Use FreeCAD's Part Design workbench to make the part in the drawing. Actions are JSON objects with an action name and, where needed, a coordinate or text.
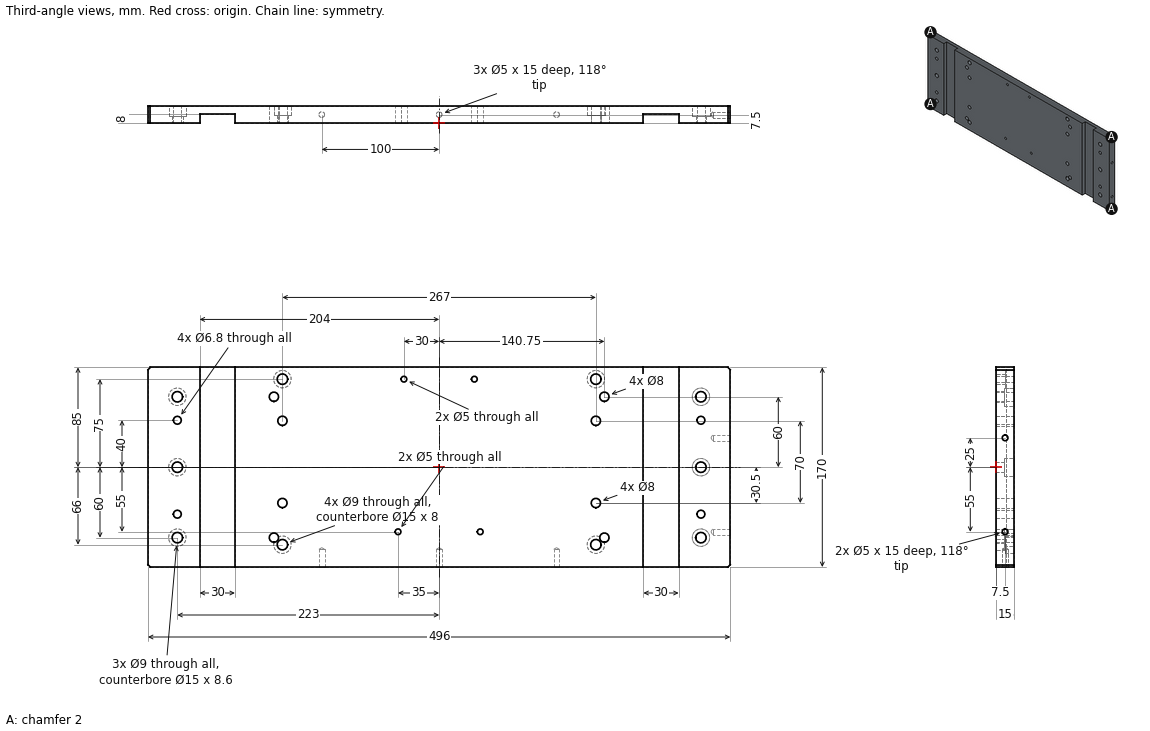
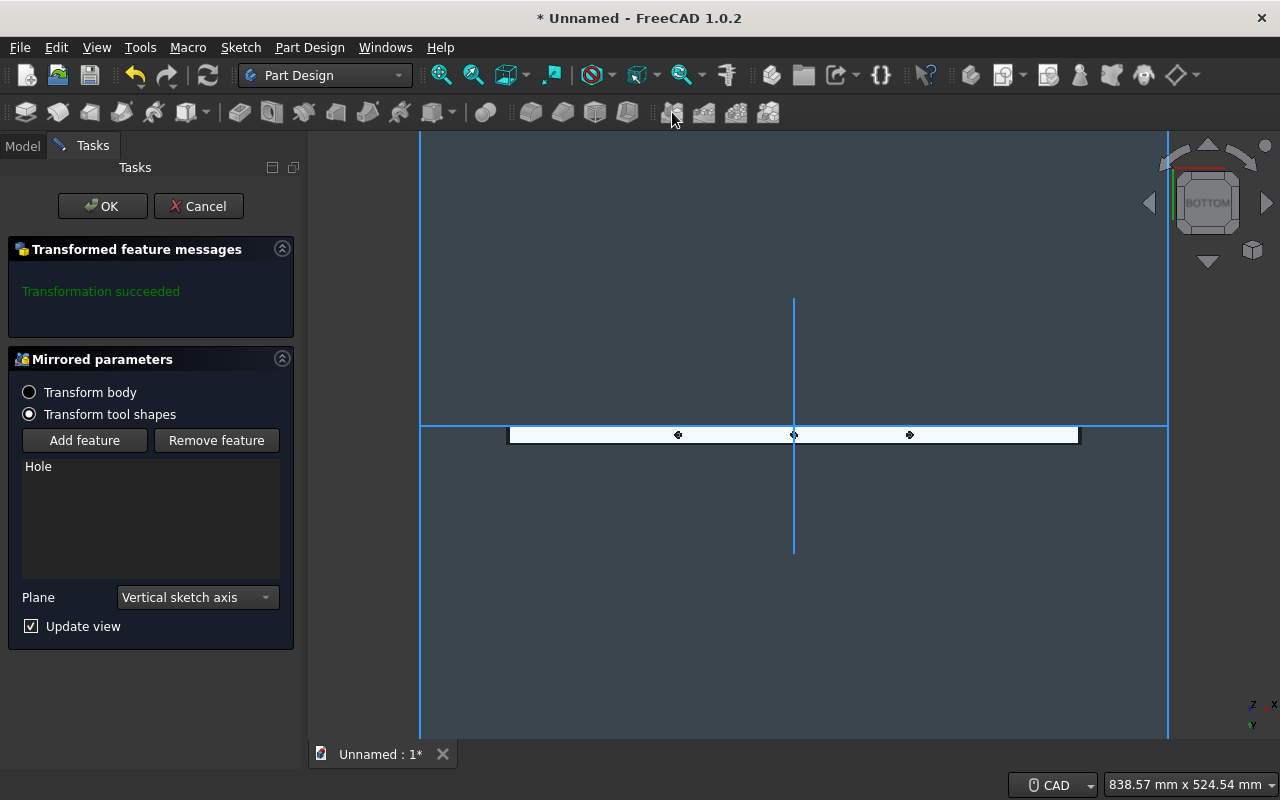
{"action": "left_click", "coordinate": [198, 598]}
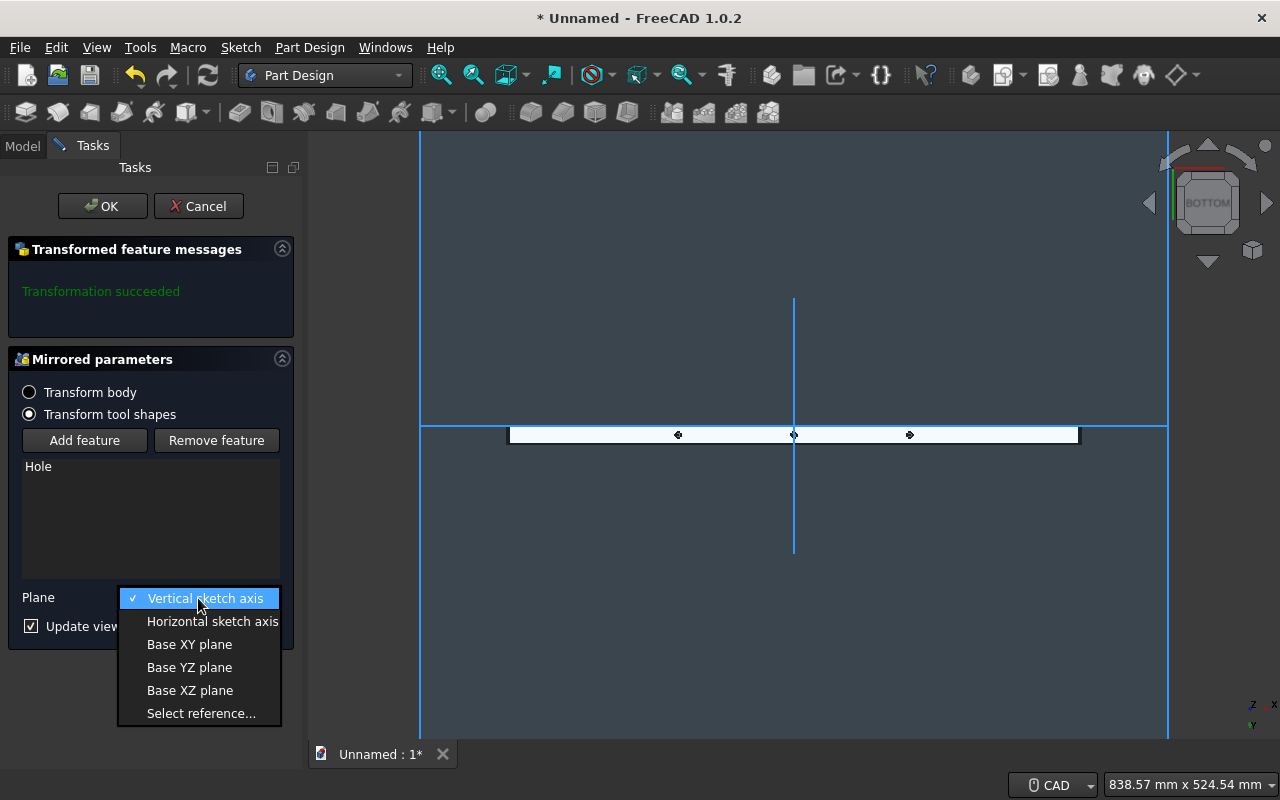
{"action": "left_click", "coordinate": [198, 668]}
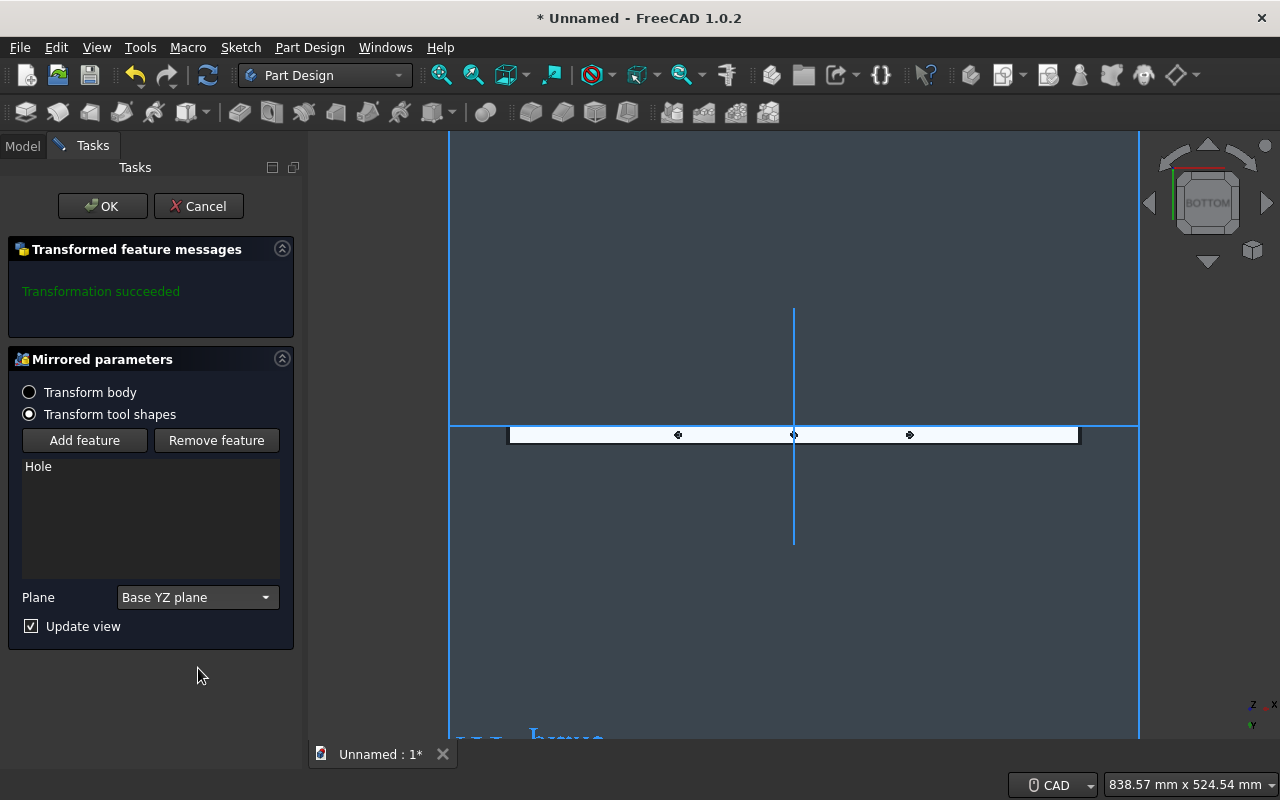
{"action": "left_click", "coordinate": [103, 206]}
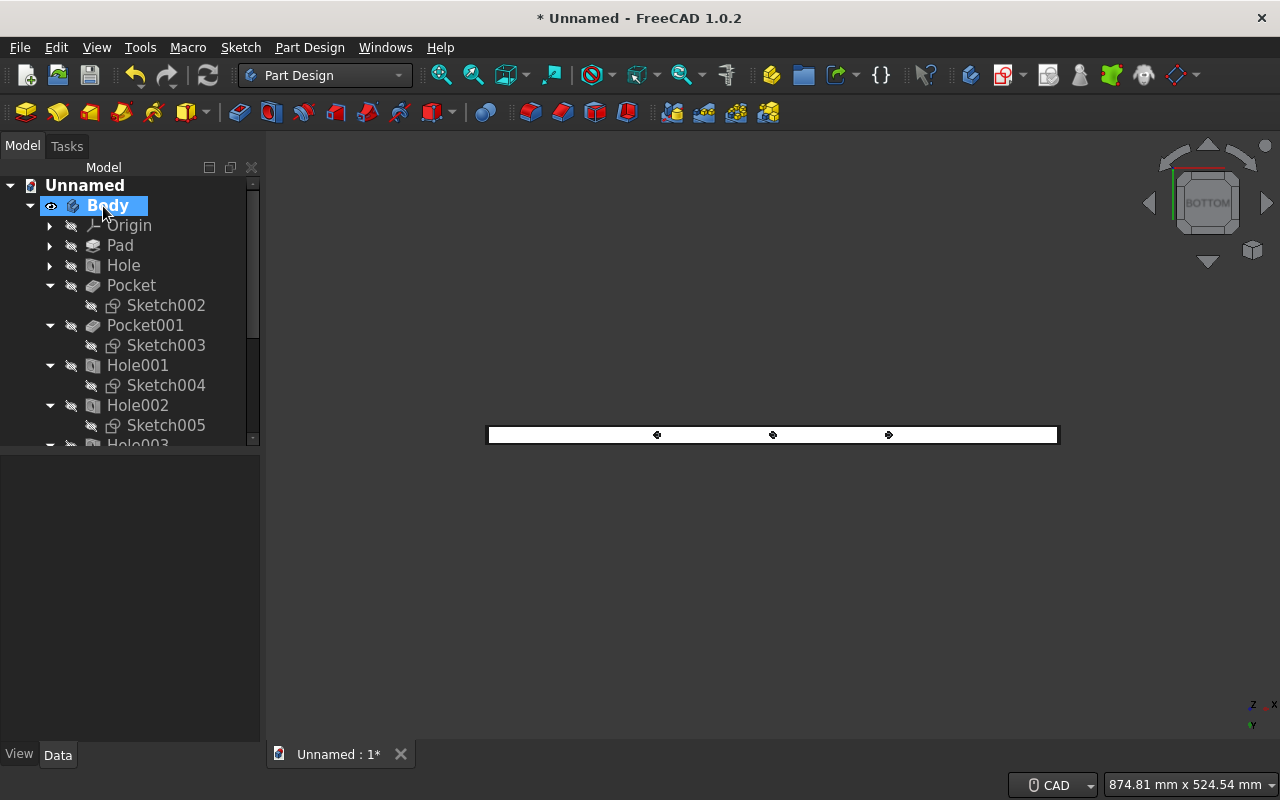
{"action": "key", "text": "0"}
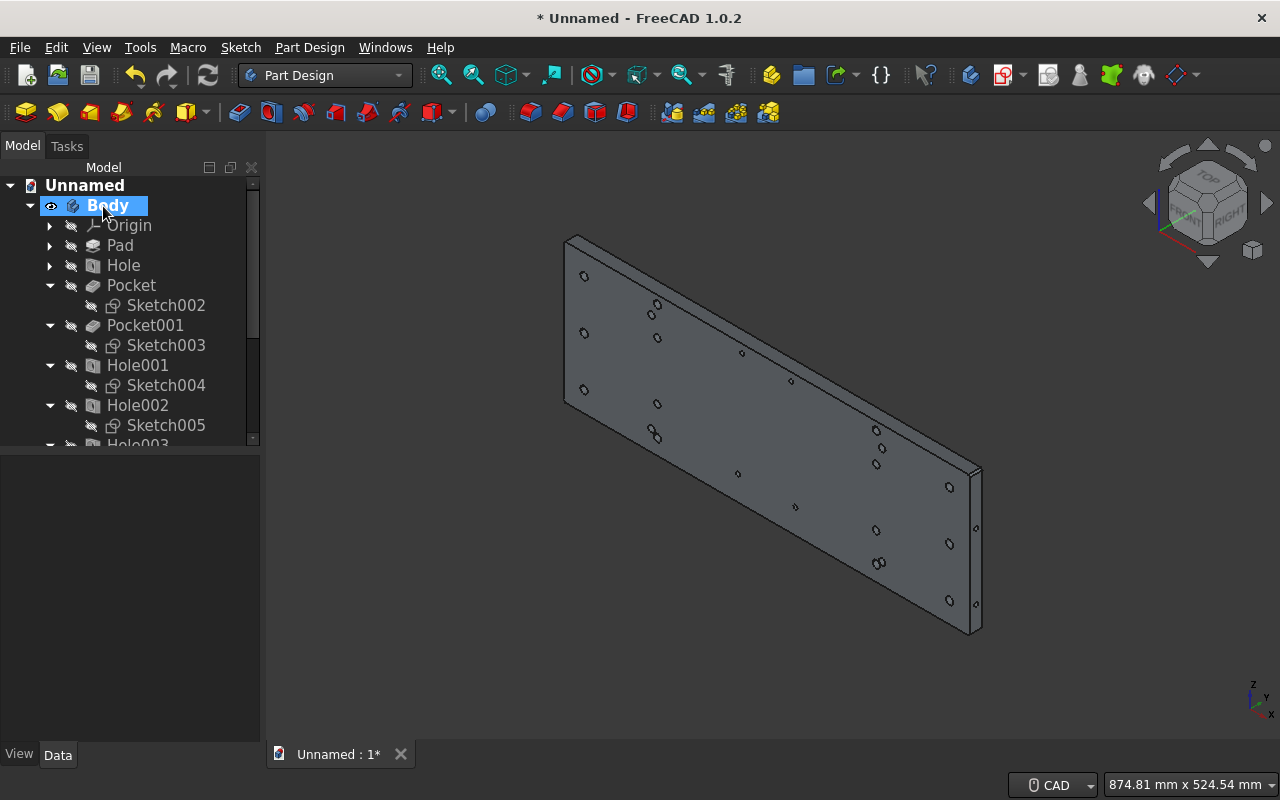
{"action": "left_click", "coordinate": [825, 471]}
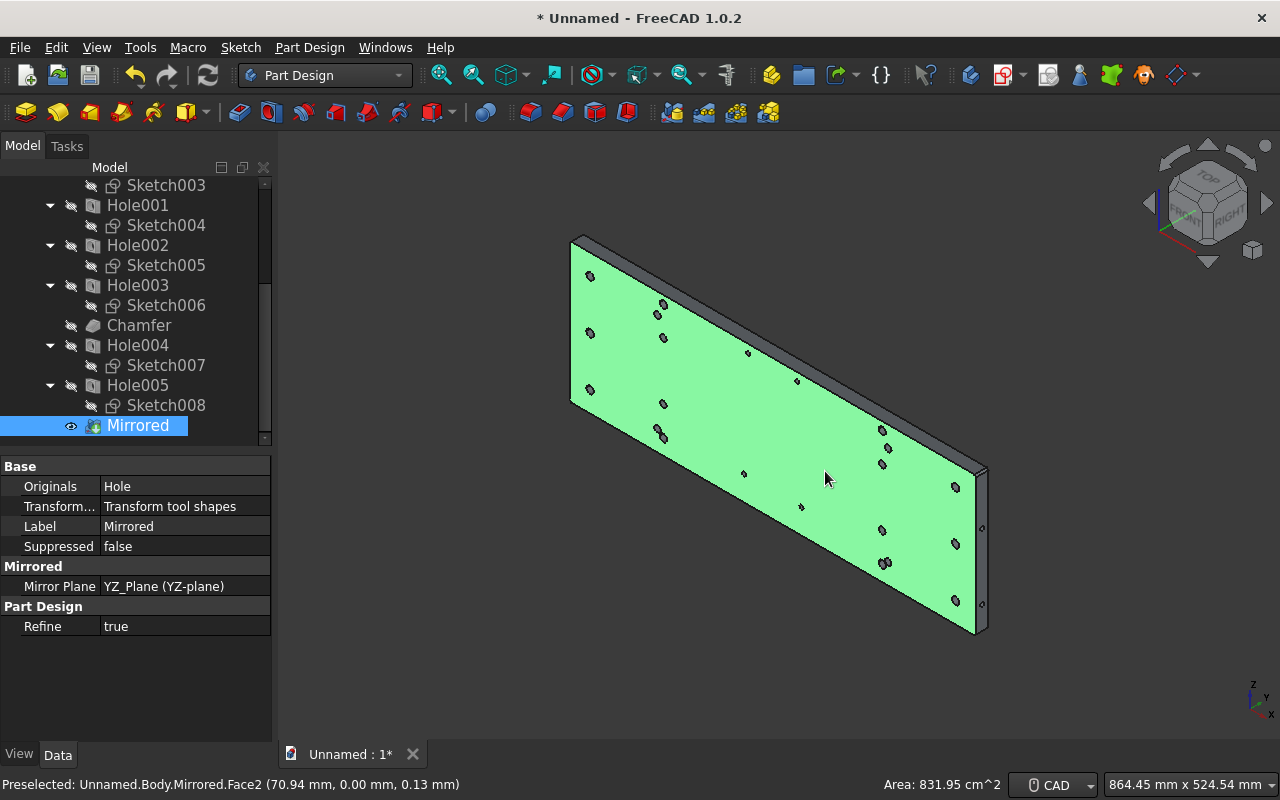
{"action": "left_click", "coordinate": [1004, 76]}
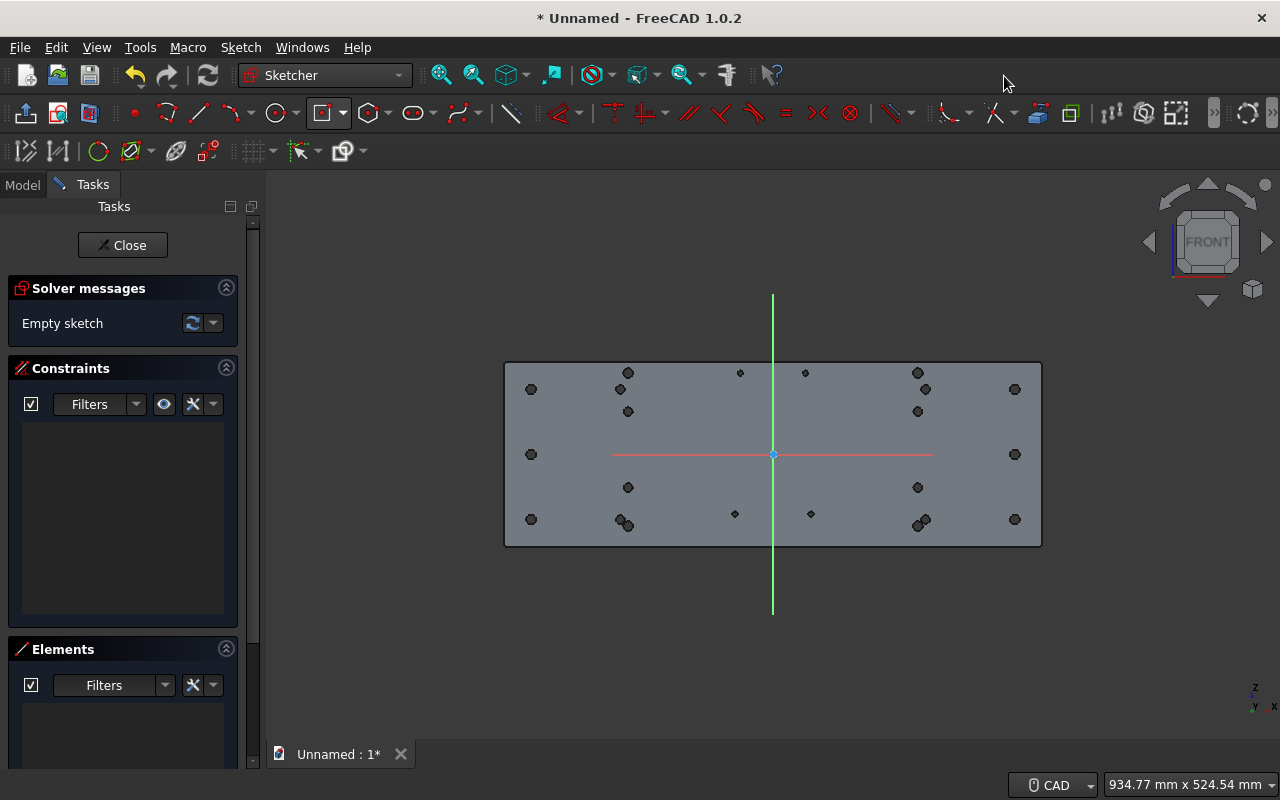
{"action": "left_click", "coordinate": [276, 114]}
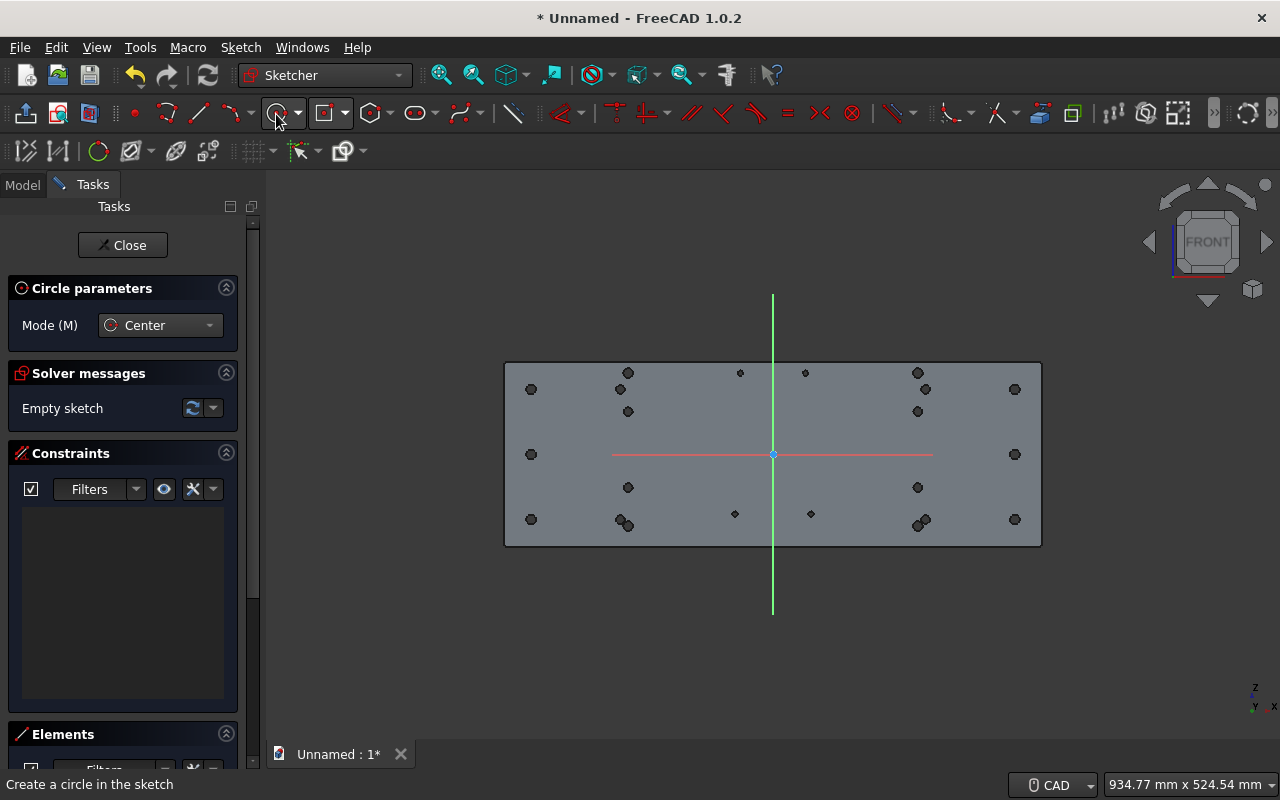
{"action": "scroll", "coordinate": [531, 411], "scroll_direction": "up", "scroll_amount": 10}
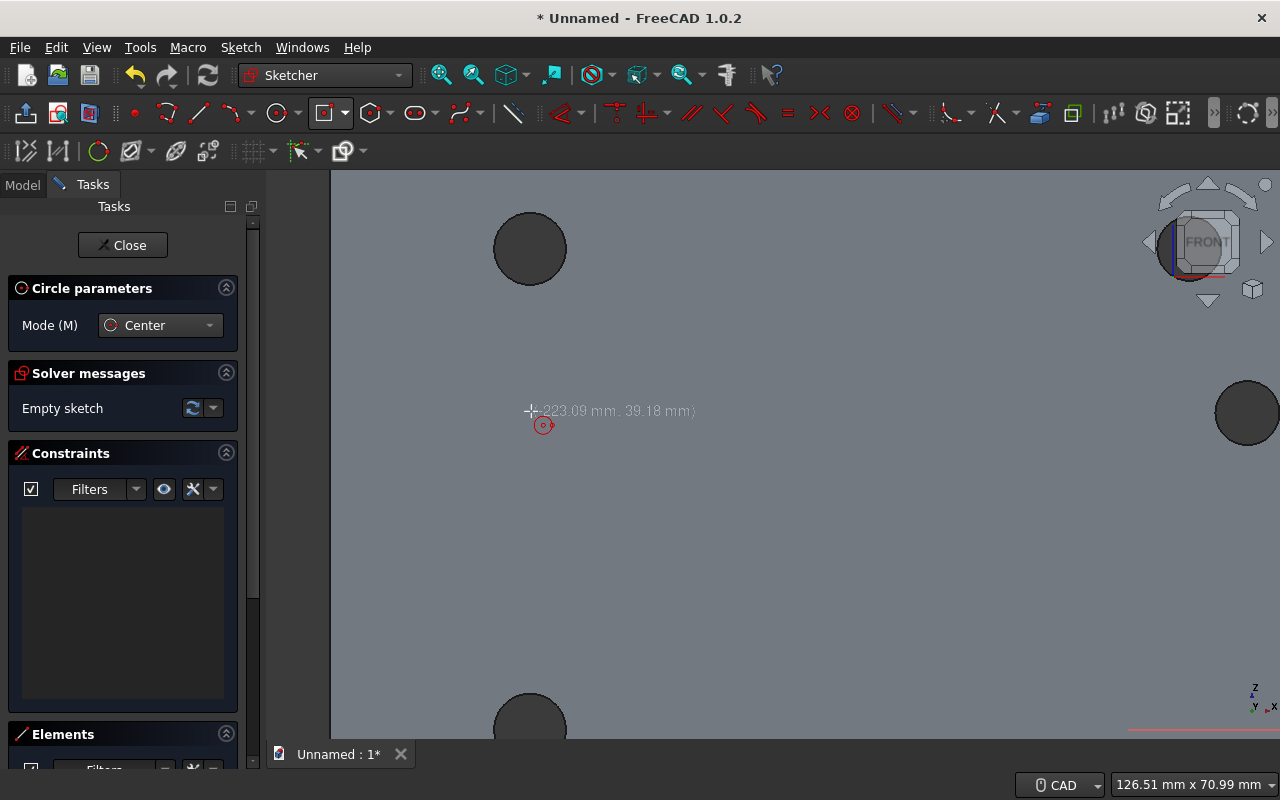
{"action": "scroll", "coordinate": [385, 400], "scroll_direction": "down", "scroll_amount": 9}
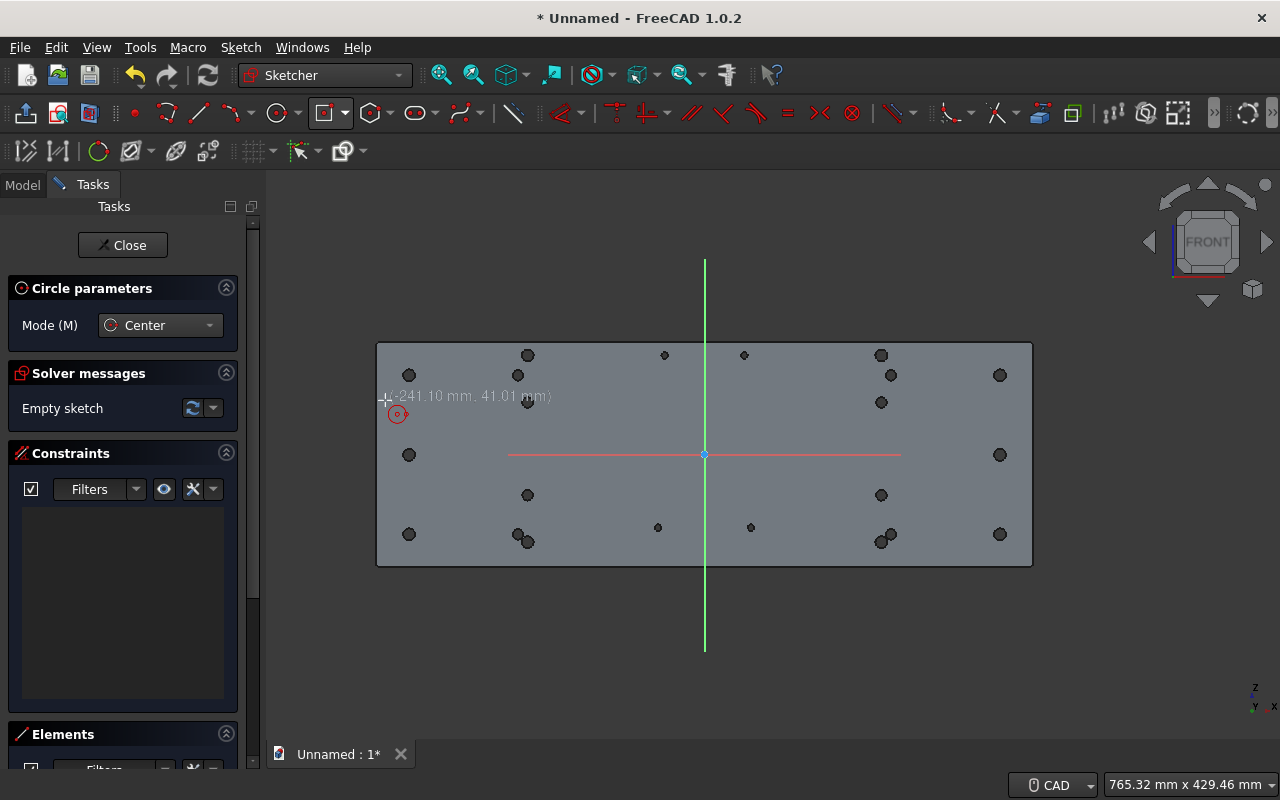
{"action": "left_click", "coordinate": [409, 402]}
{"action": "mouse_move", "coordinate": [412, 399]}